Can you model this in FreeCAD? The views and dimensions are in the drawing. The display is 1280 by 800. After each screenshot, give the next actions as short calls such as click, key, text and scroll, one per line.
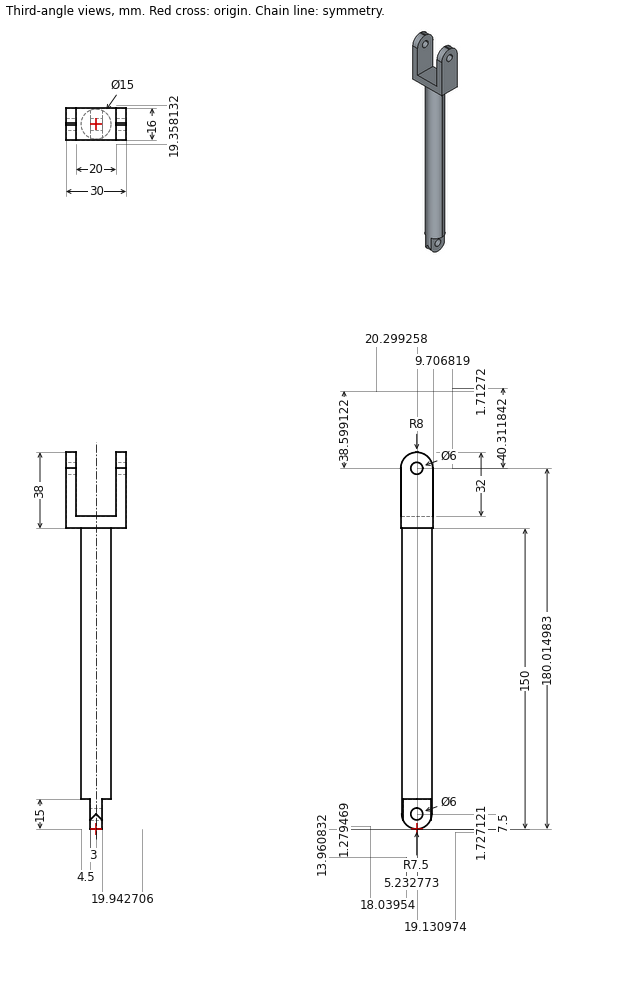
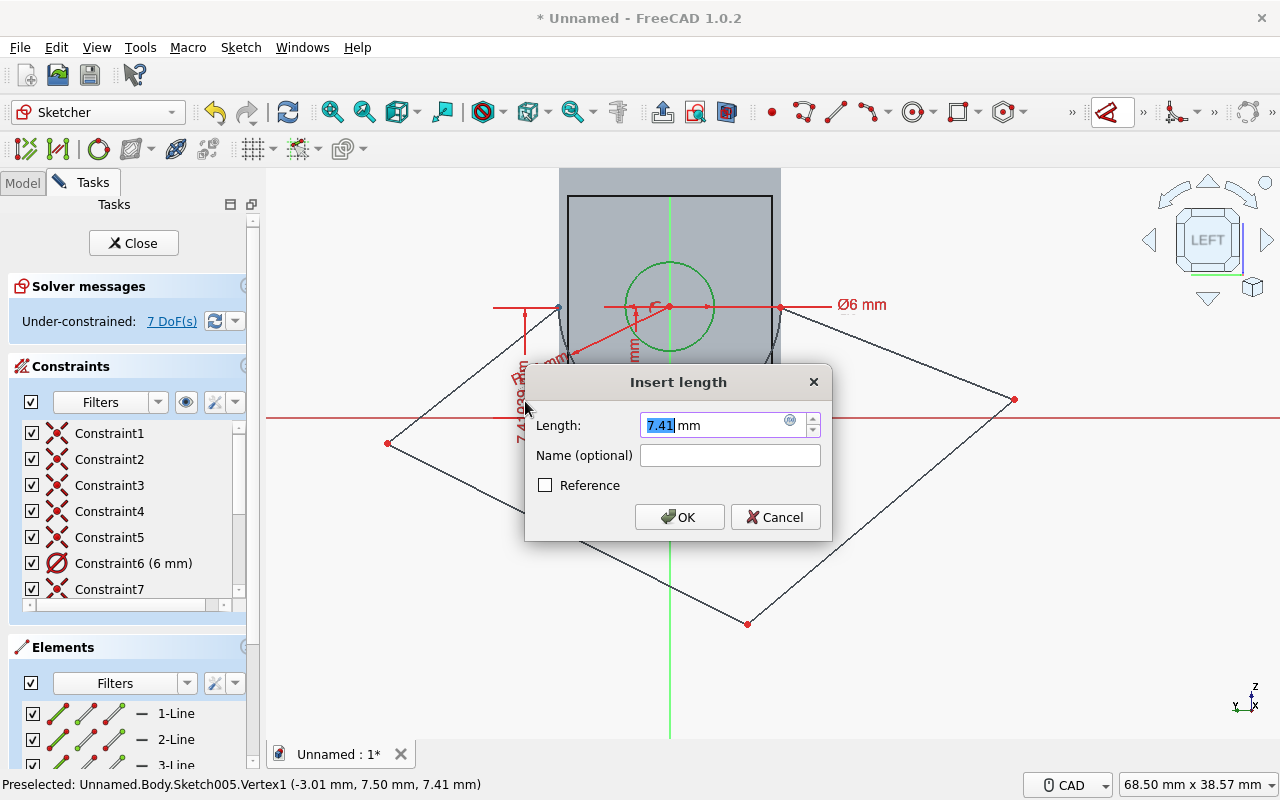
text(7.5)
key(Return)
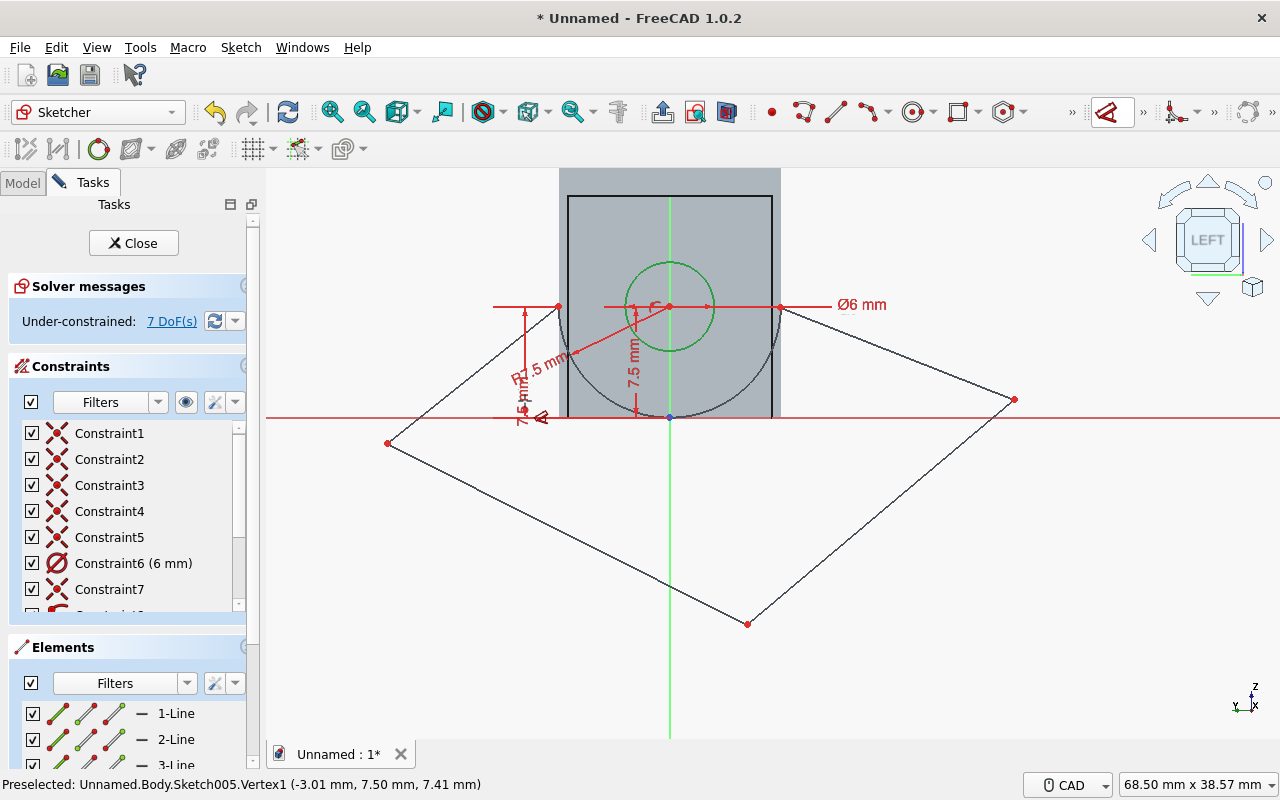
click(781, 308)
click(815, 363)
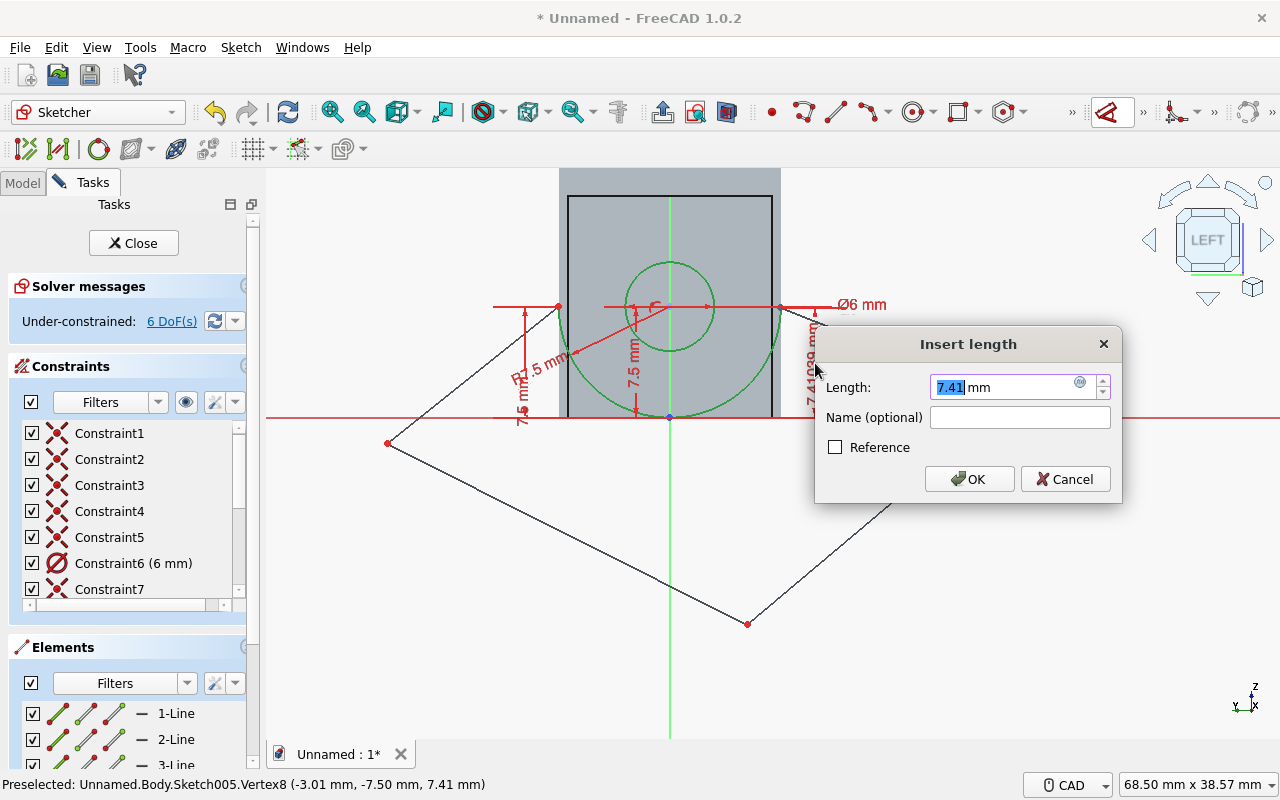
text(7.5)
key(Return)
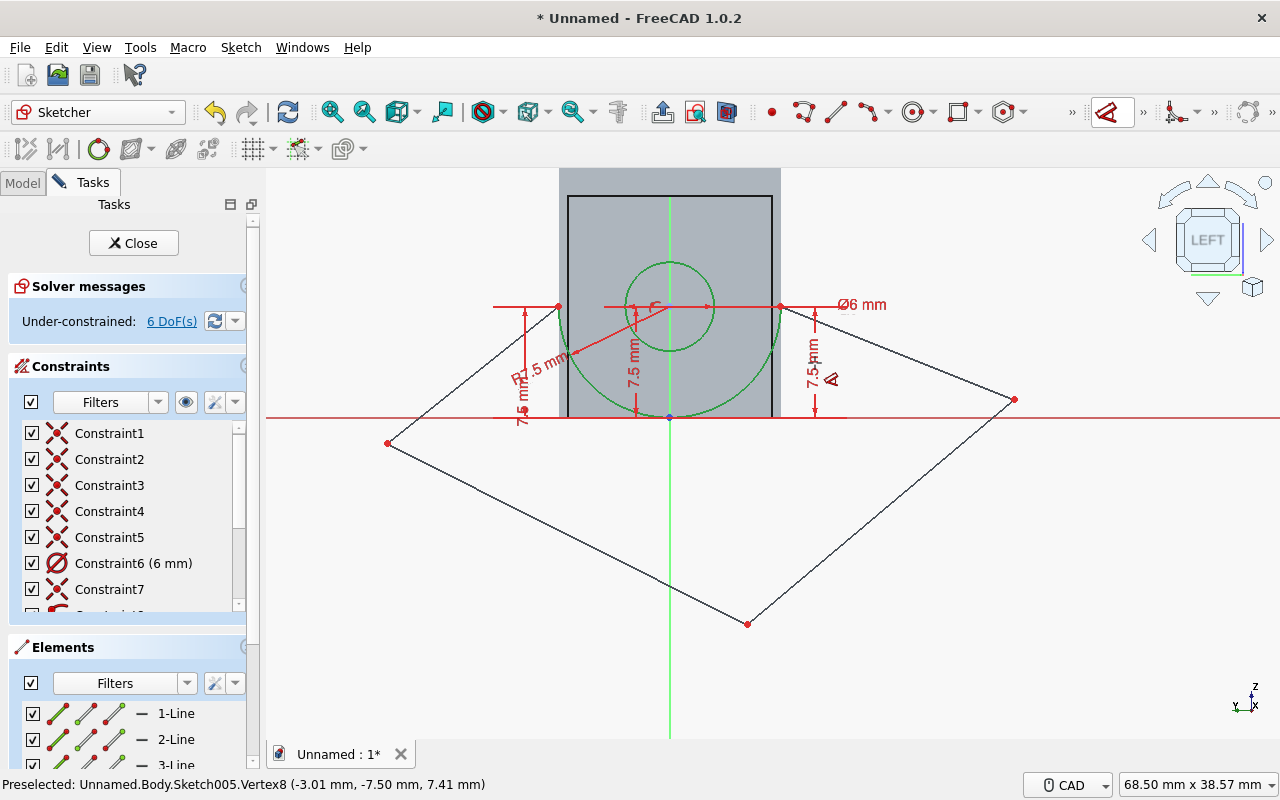
scroll(387, 444, up, 3)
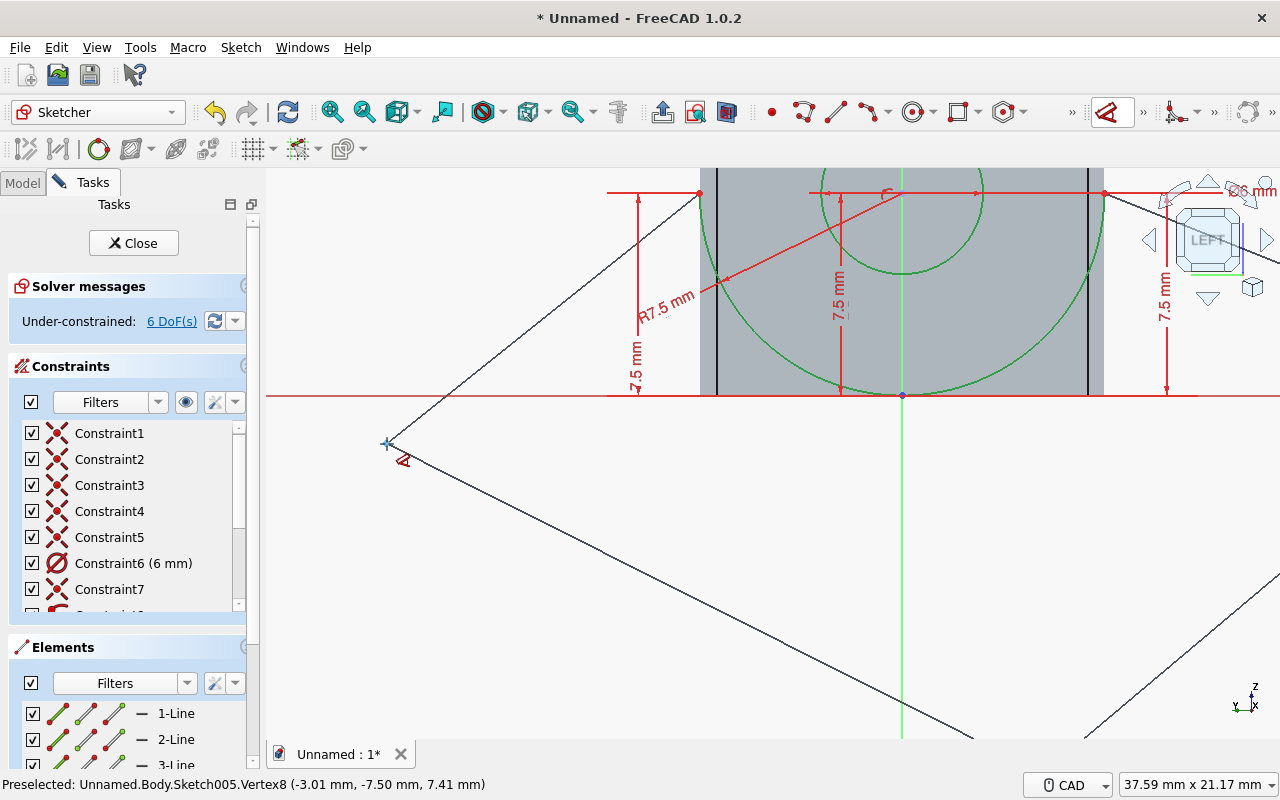
click(387, 444)
click(353, 420)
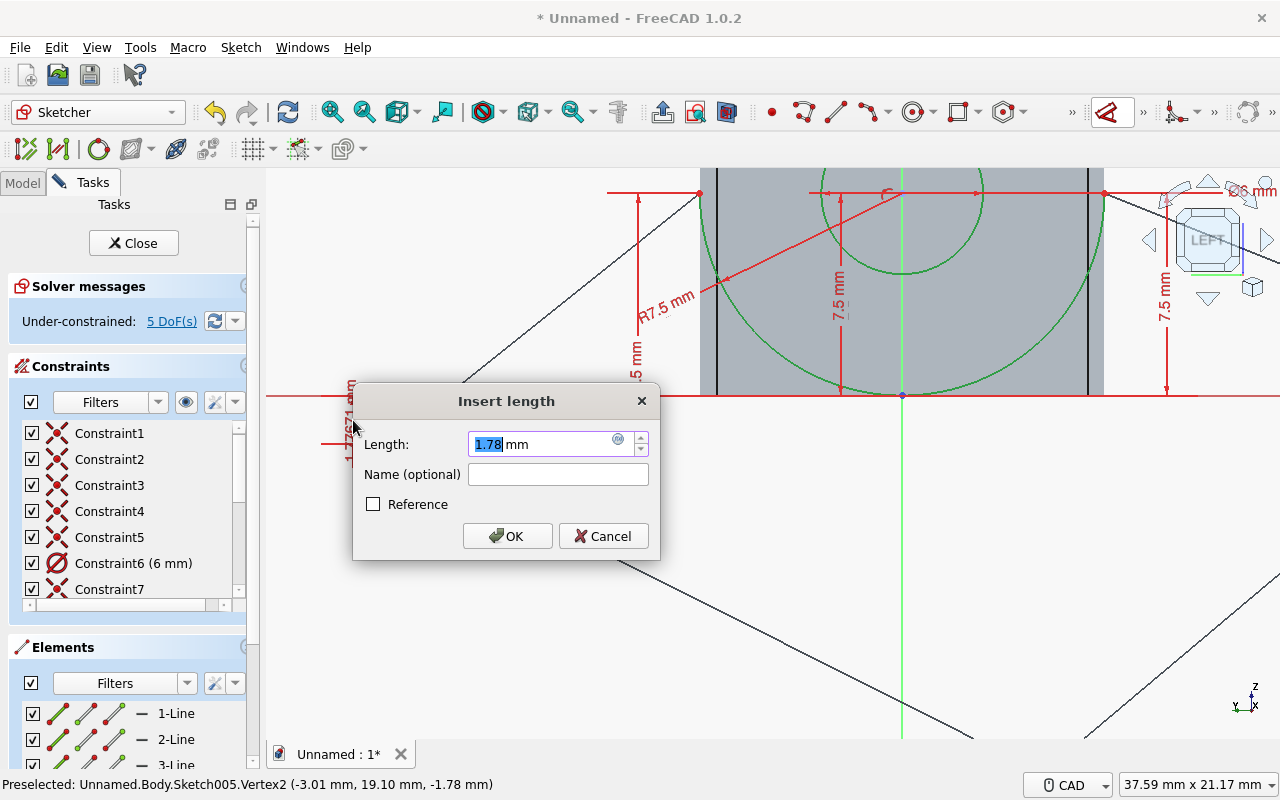
text(1.727121)
key(Return)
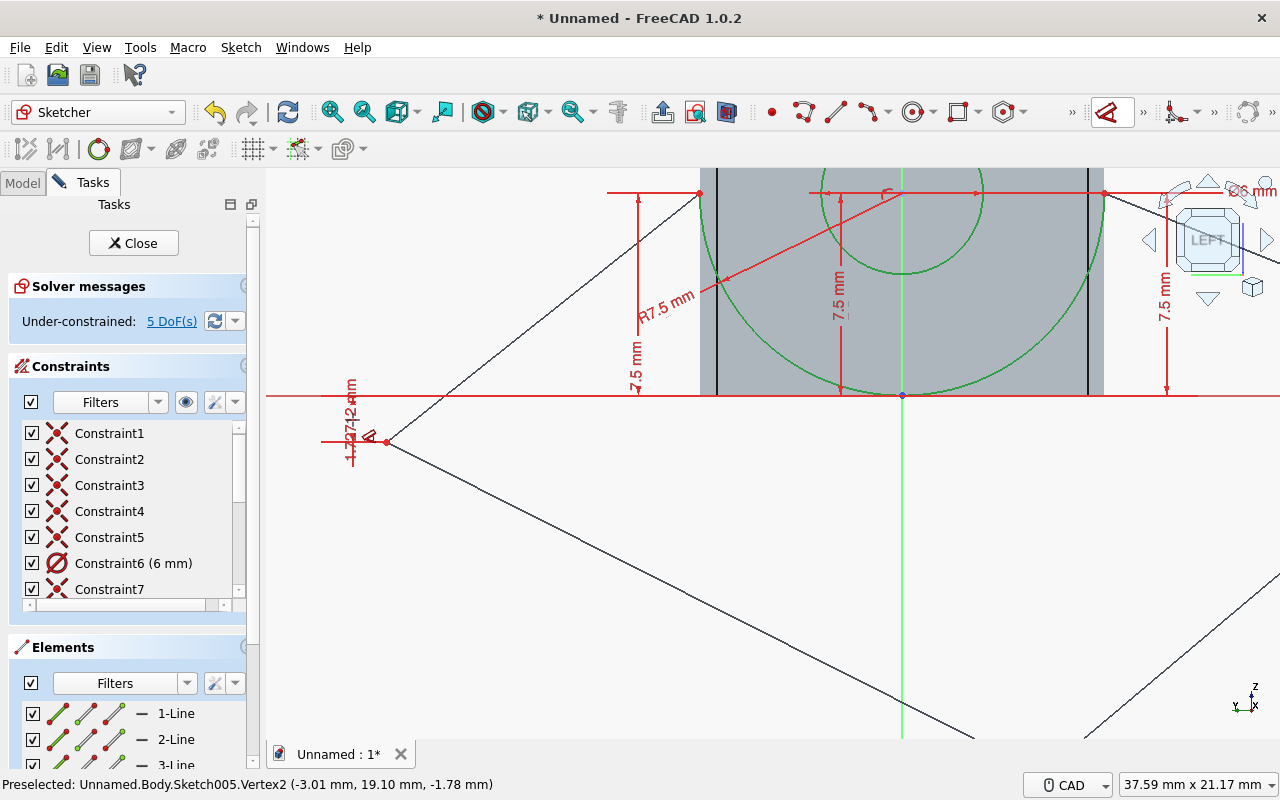
scroll(396, 467, down, 3)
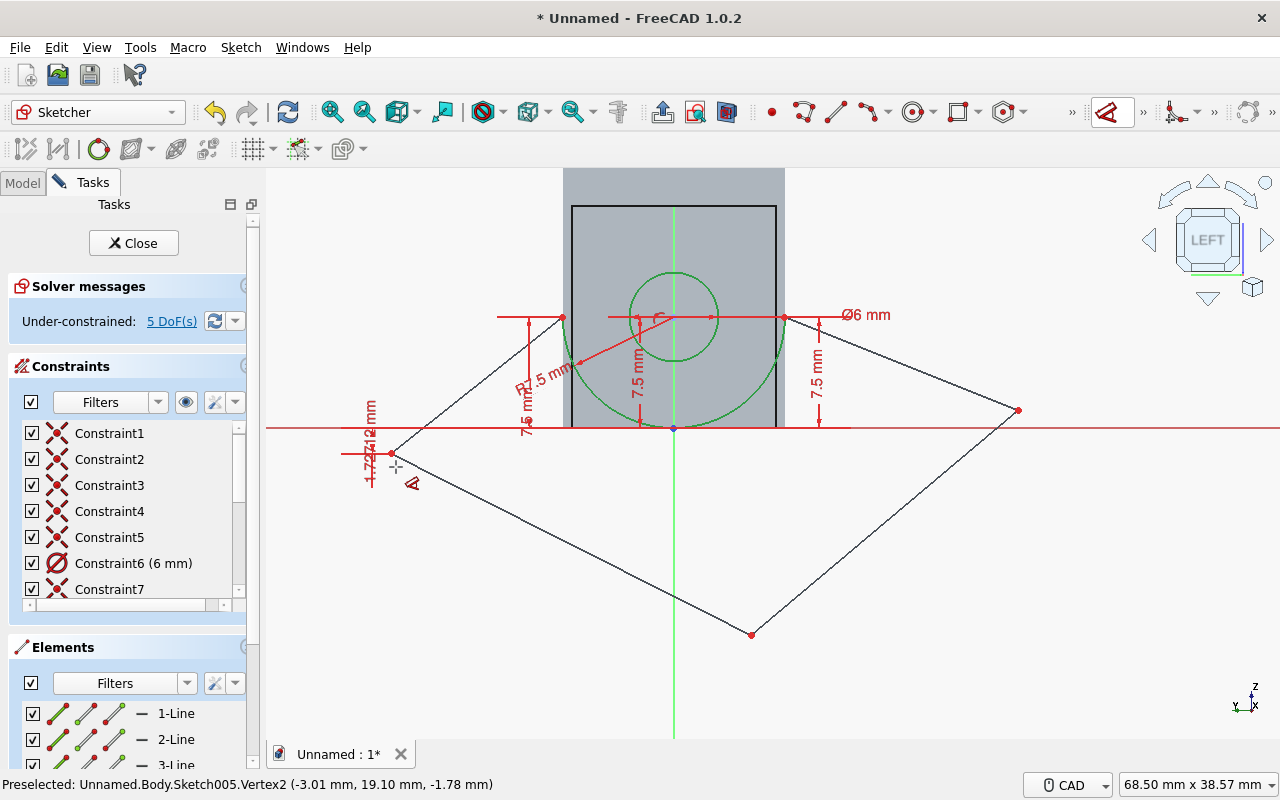
click(751, 635)
click(712, 669)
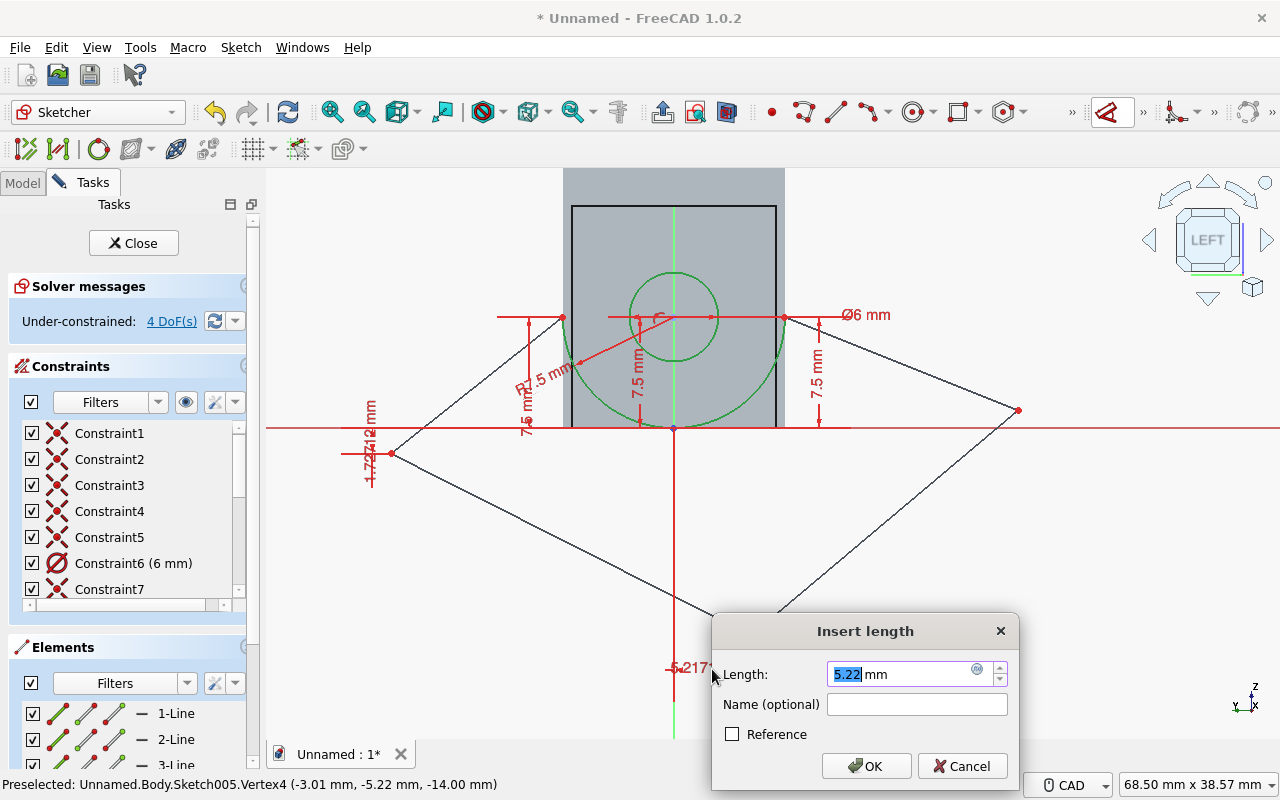
text(5.232773)
key(Return)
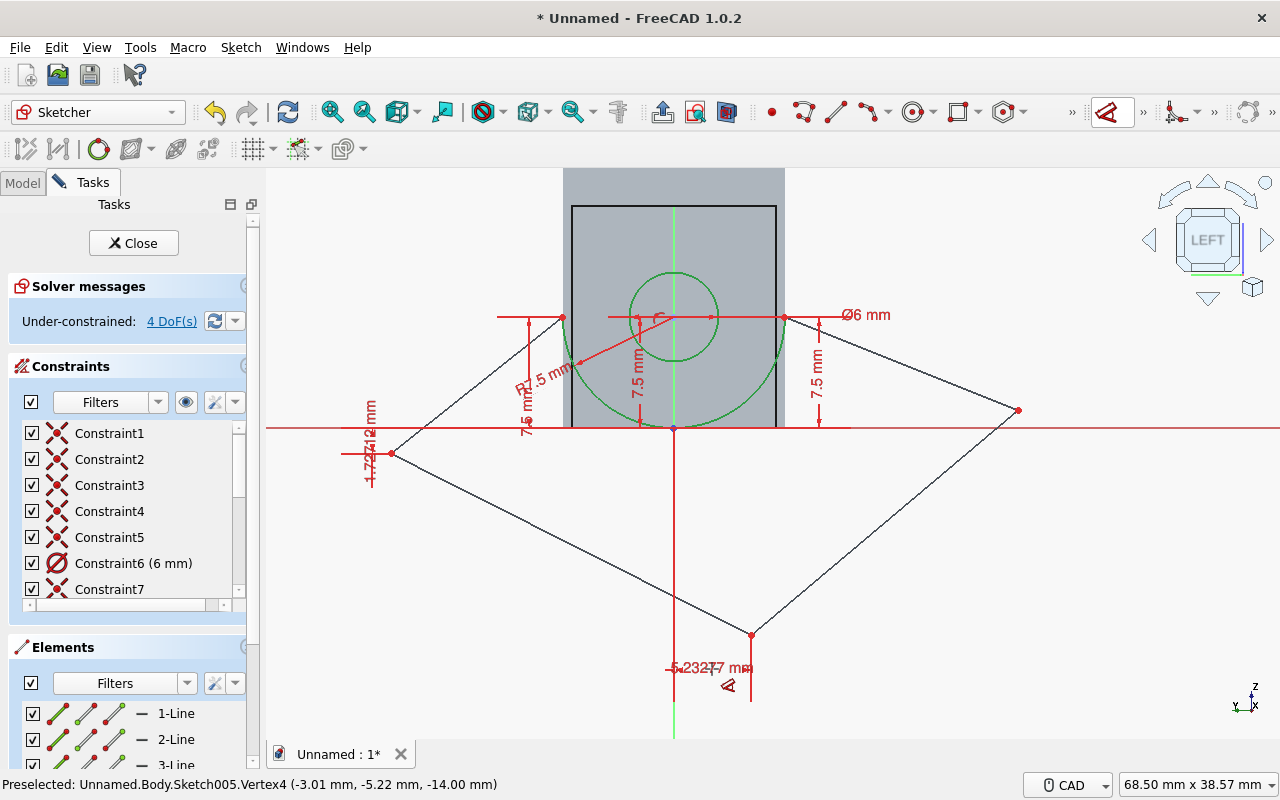
scroll(1018, 410, up, 4)